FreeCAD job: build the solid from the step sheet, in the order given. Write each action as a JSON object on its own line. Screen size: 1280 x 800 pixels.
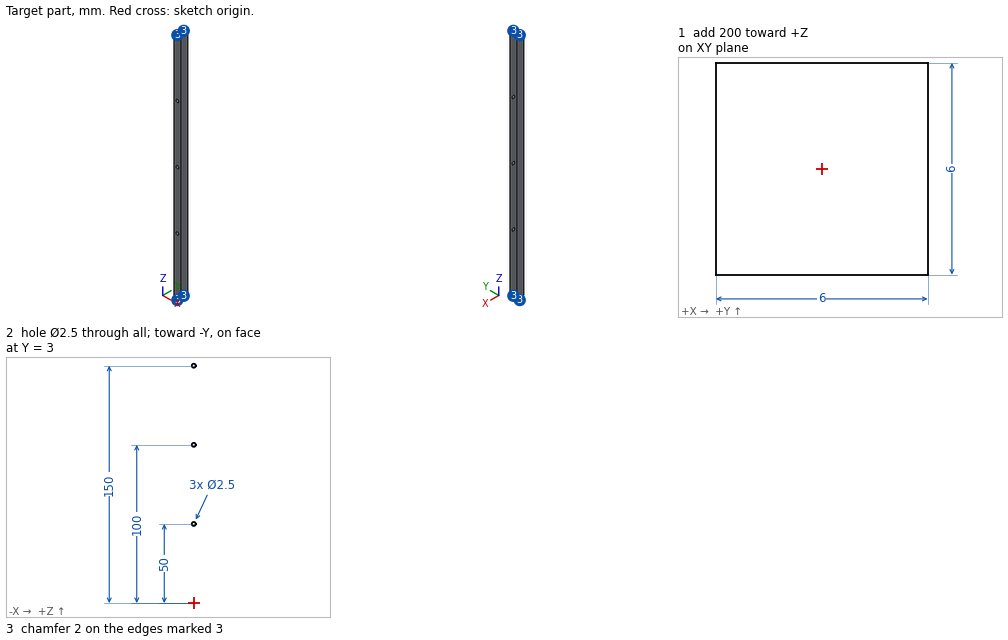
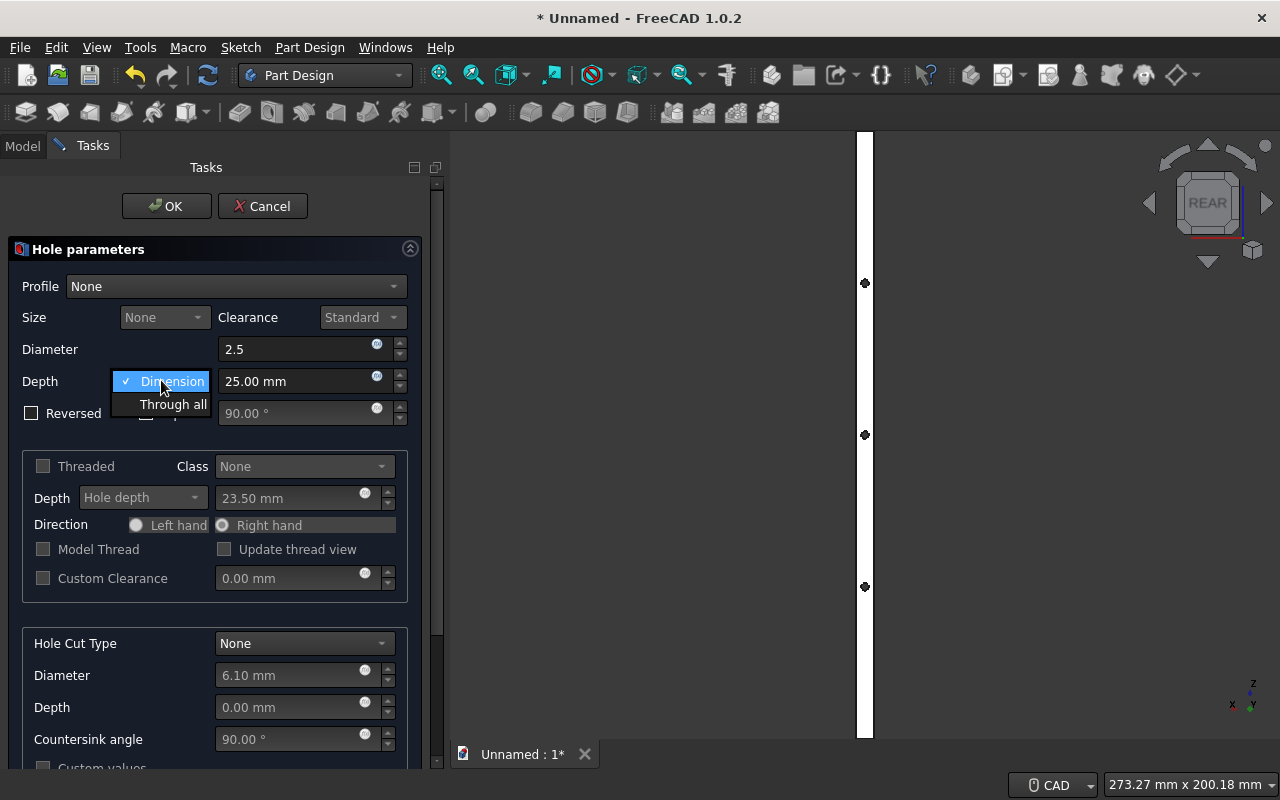
{"action": "left_click", "coordinate": [160, 404]}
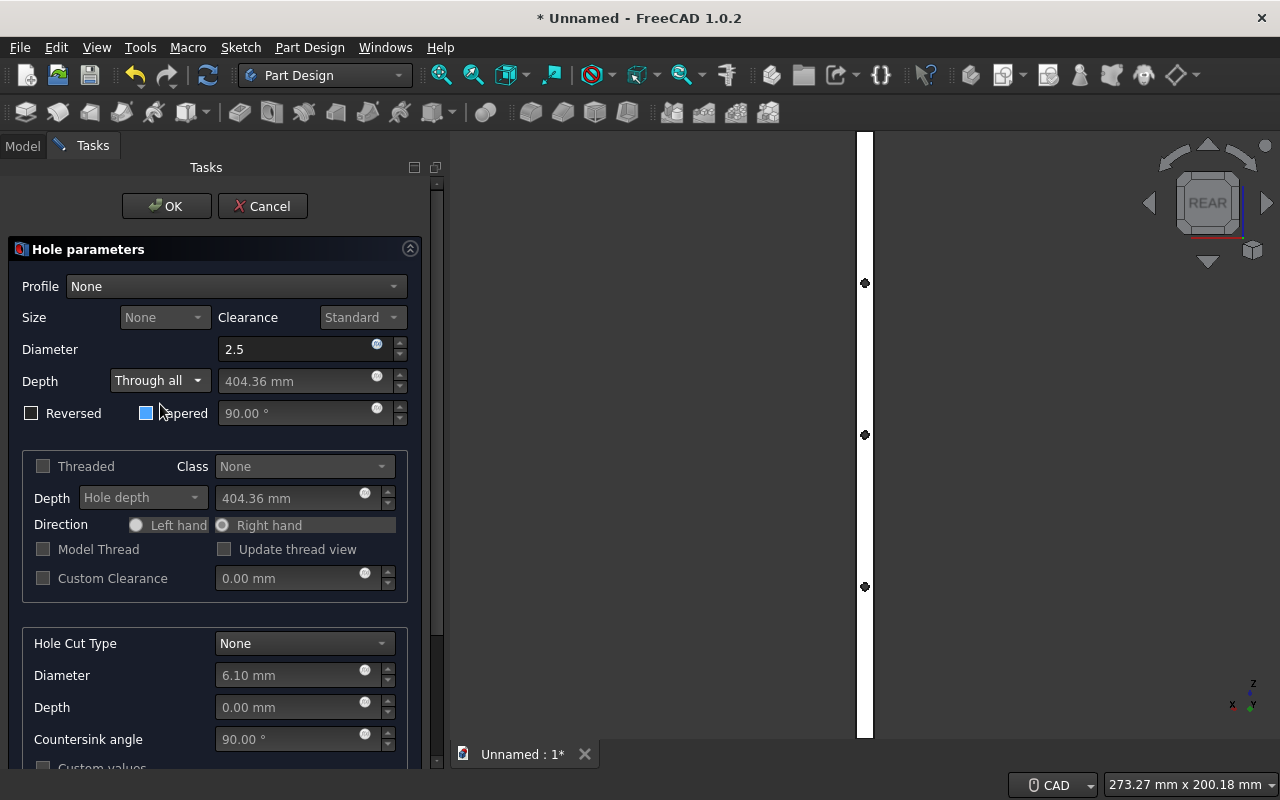
{"action": "left_click", "coordinate": [167, 206]}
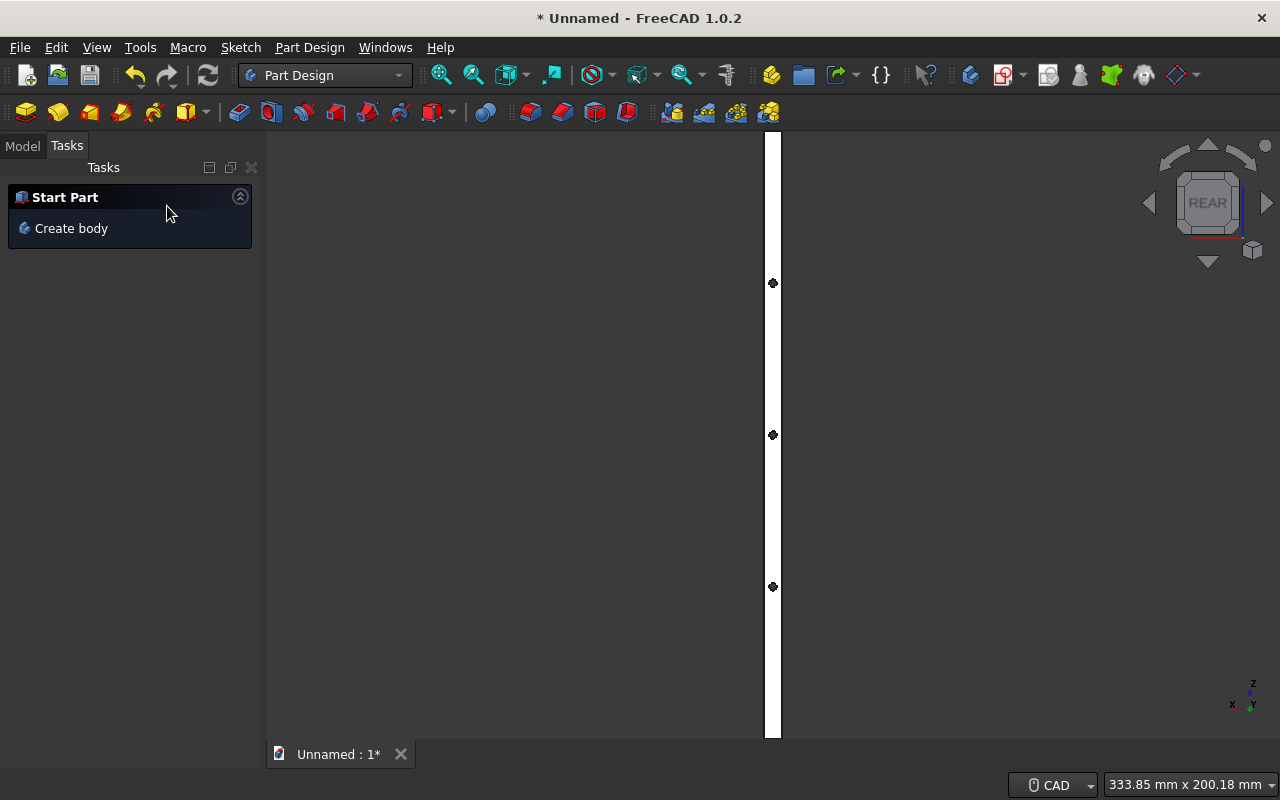
{"action": "left_click", "coordinate": [442, 76]}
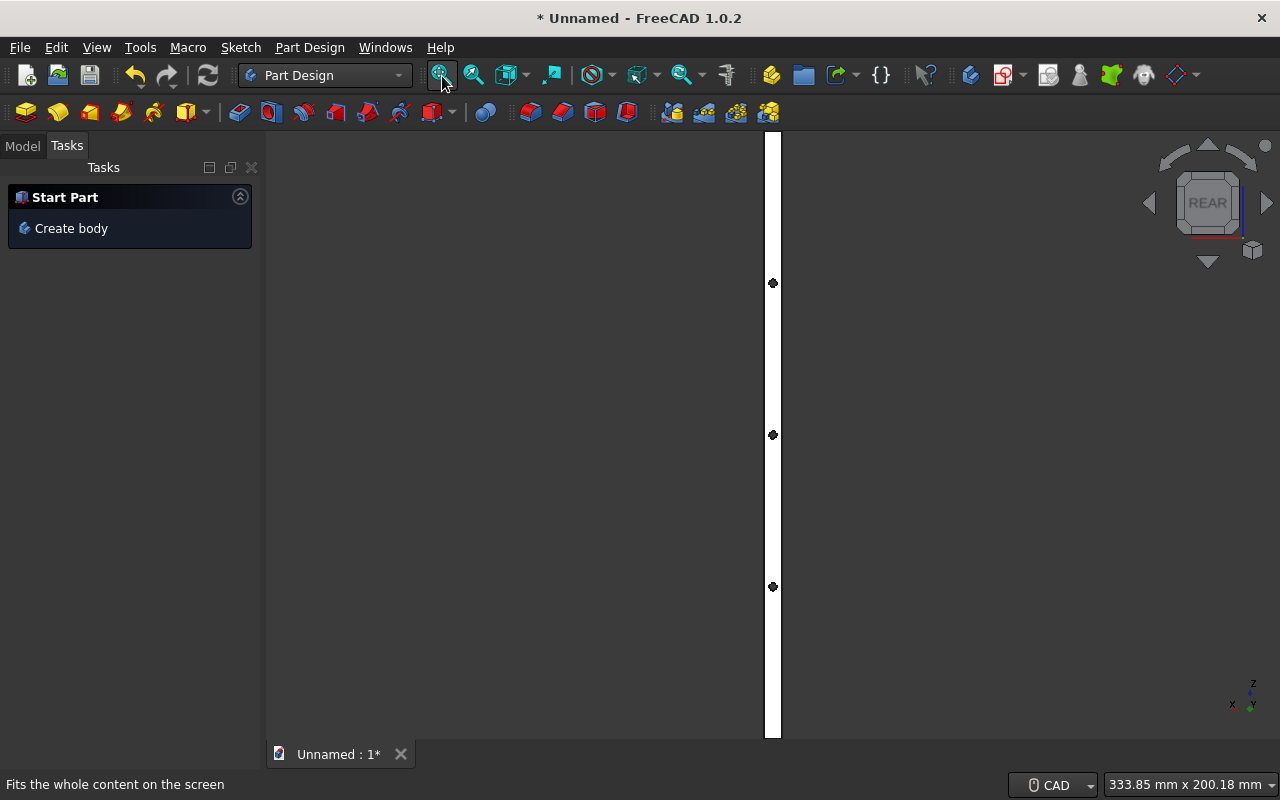
{"action": "key", "text": "0"}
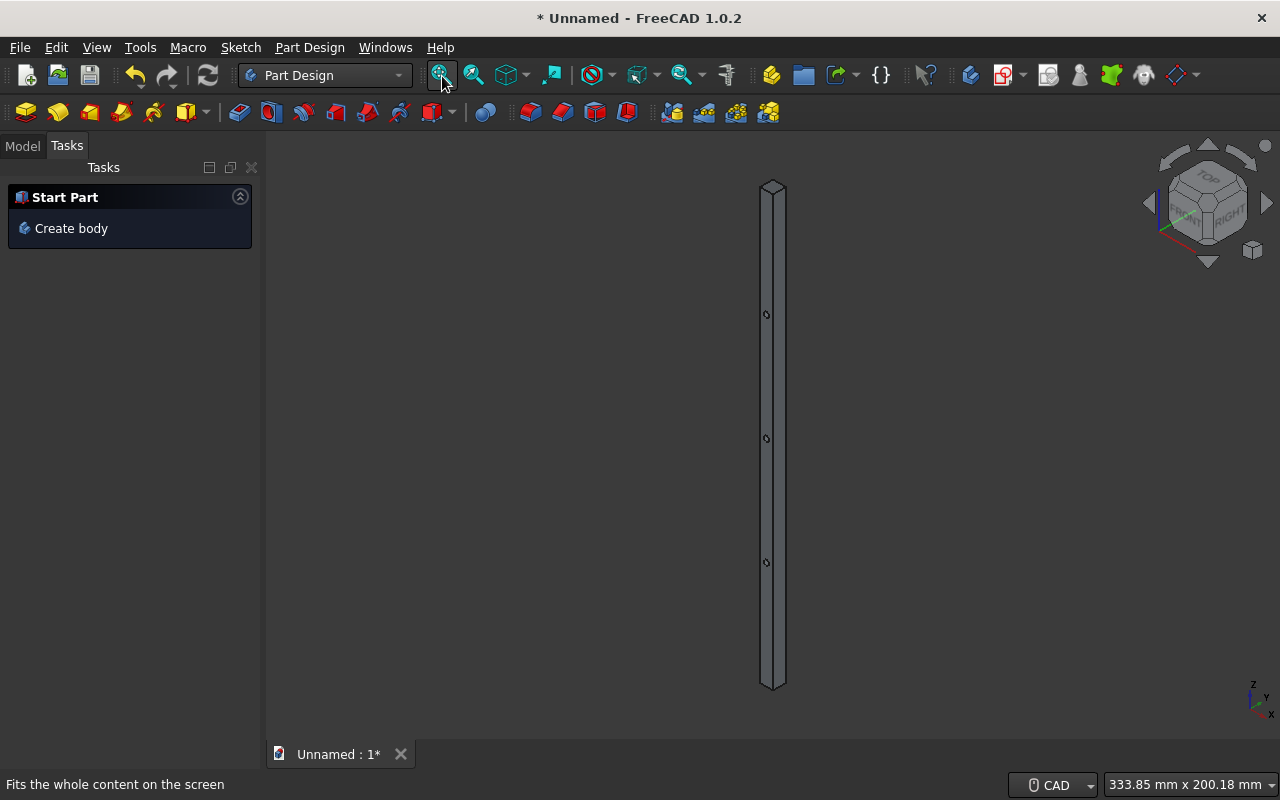
{"action": "left_click", "coordinate": [767, 190]}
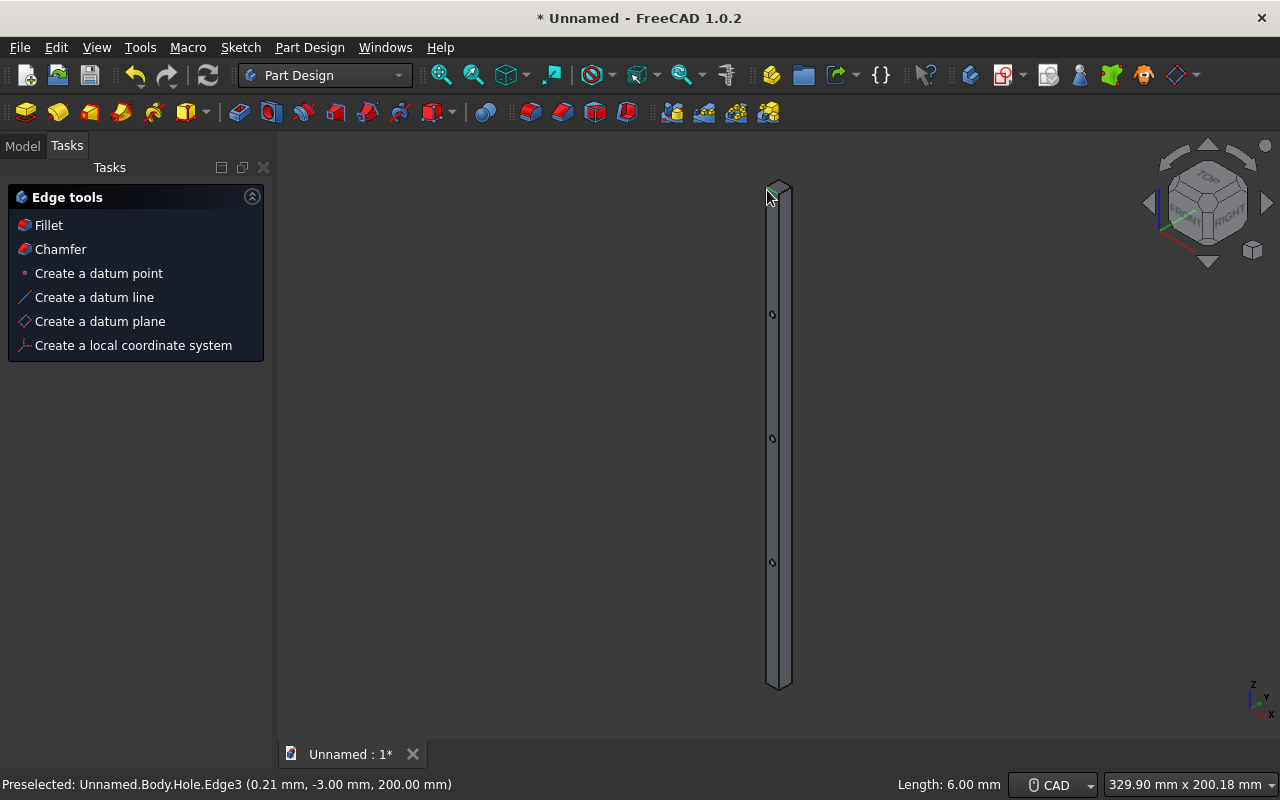
{"action": "scroll", "coordinate": [773, 686], "scroll_direction": "up", "scroll_amount": 4}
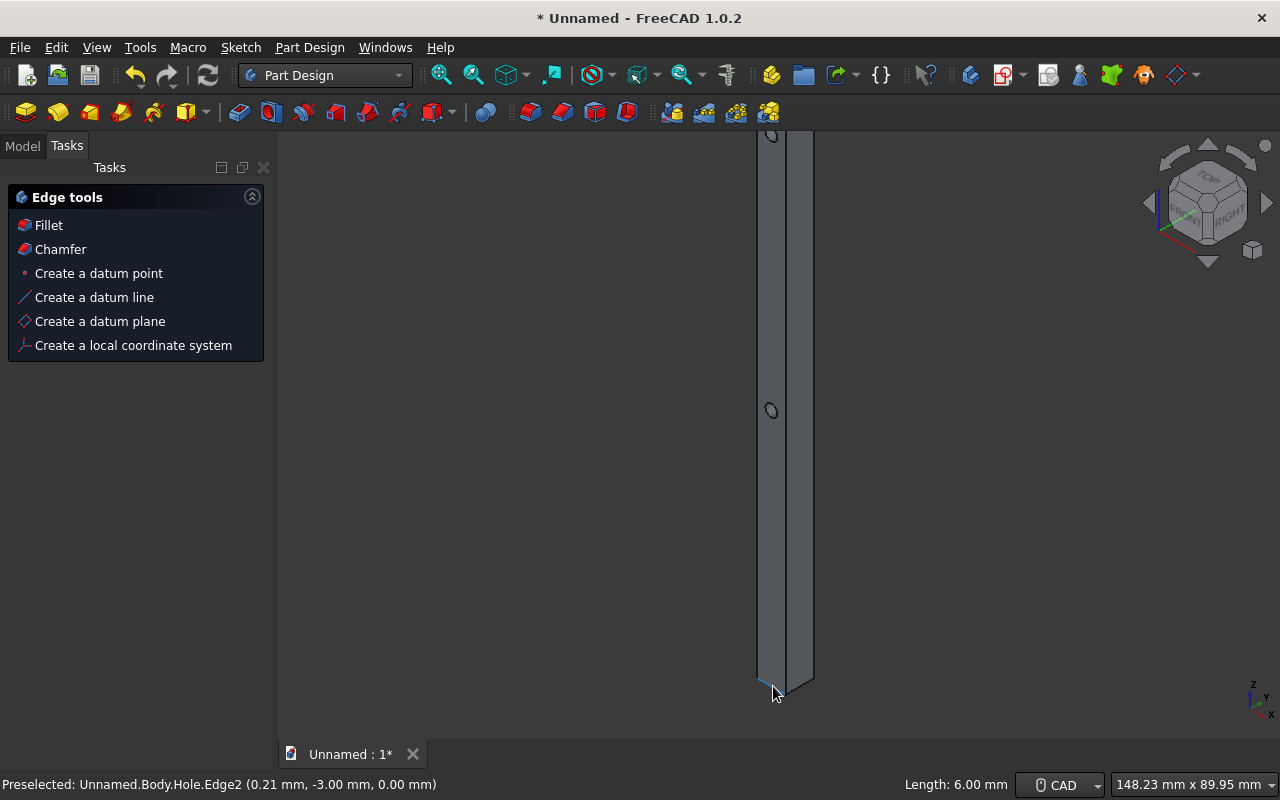
{"action": "left_click", "coordinate": [442, 76]}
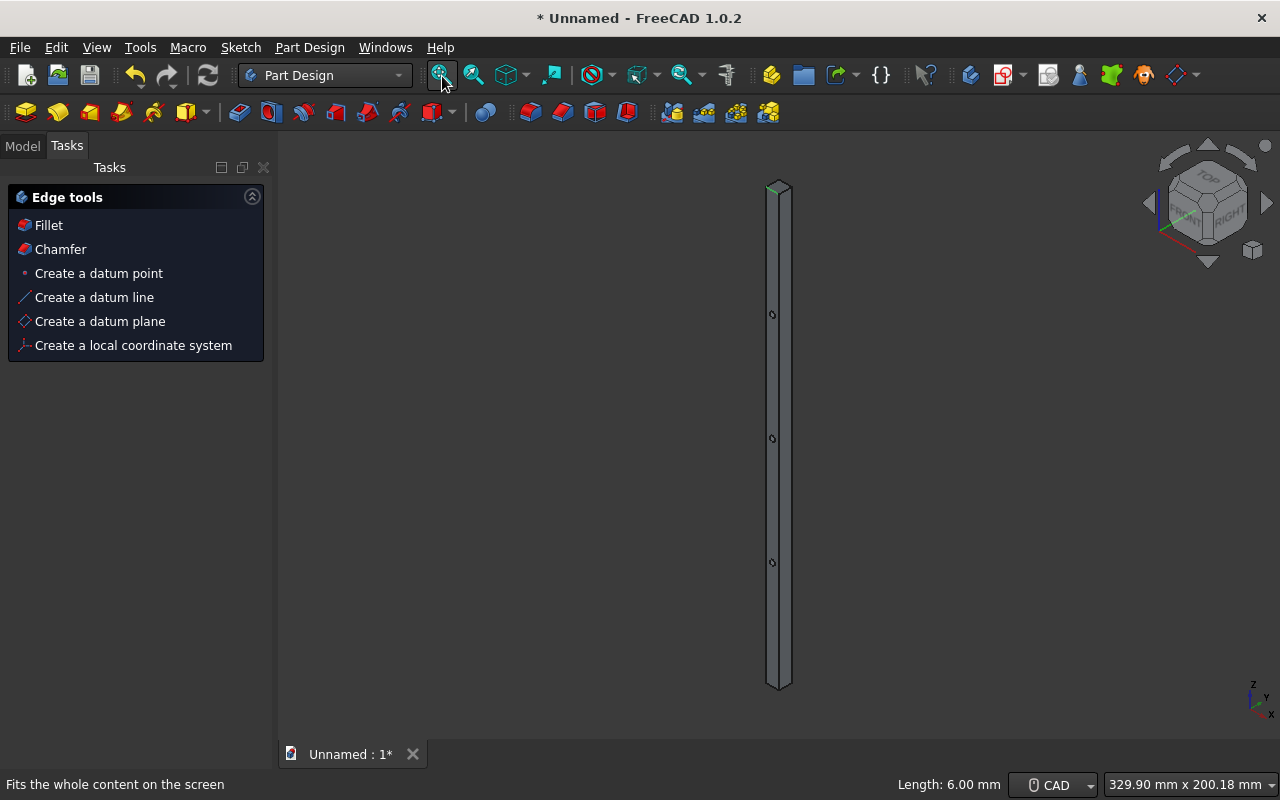
{"action": "key", "text": "2"}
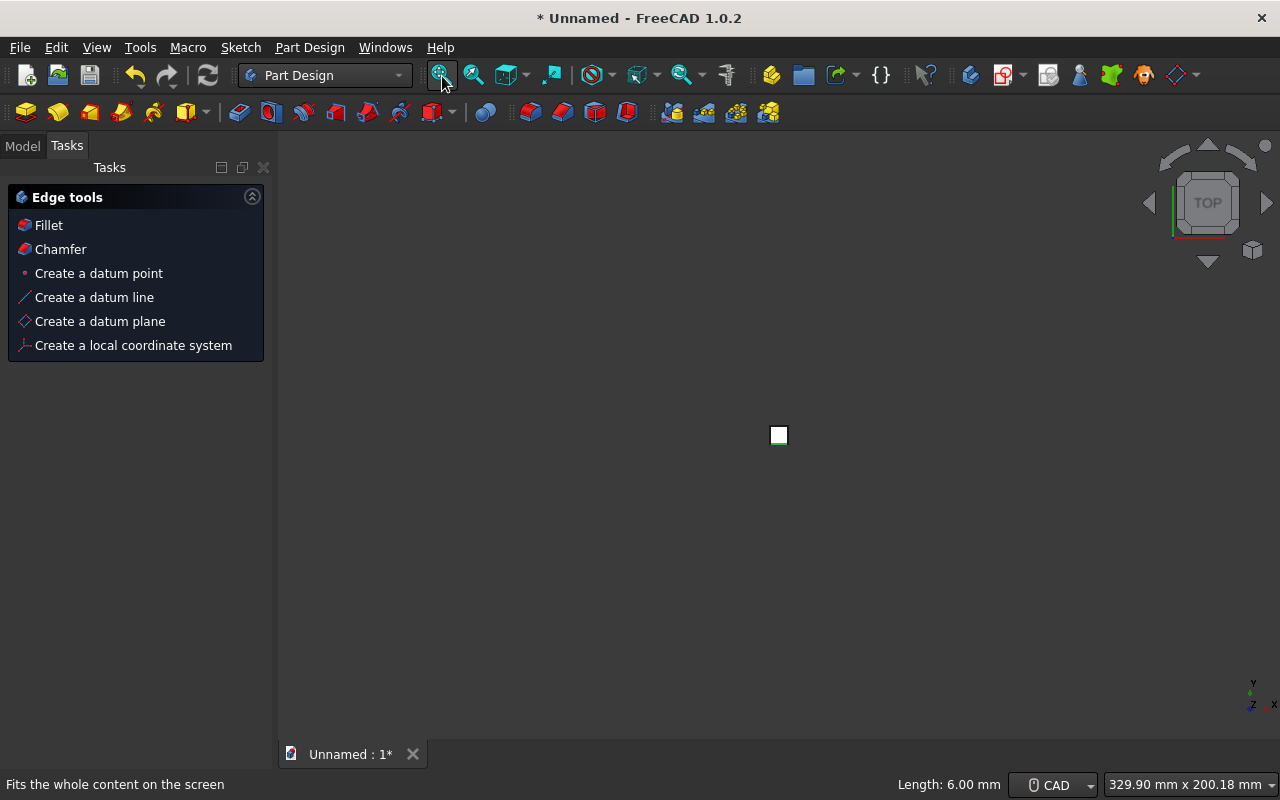
{"action": "left_click", "coordinate": [442, 76]}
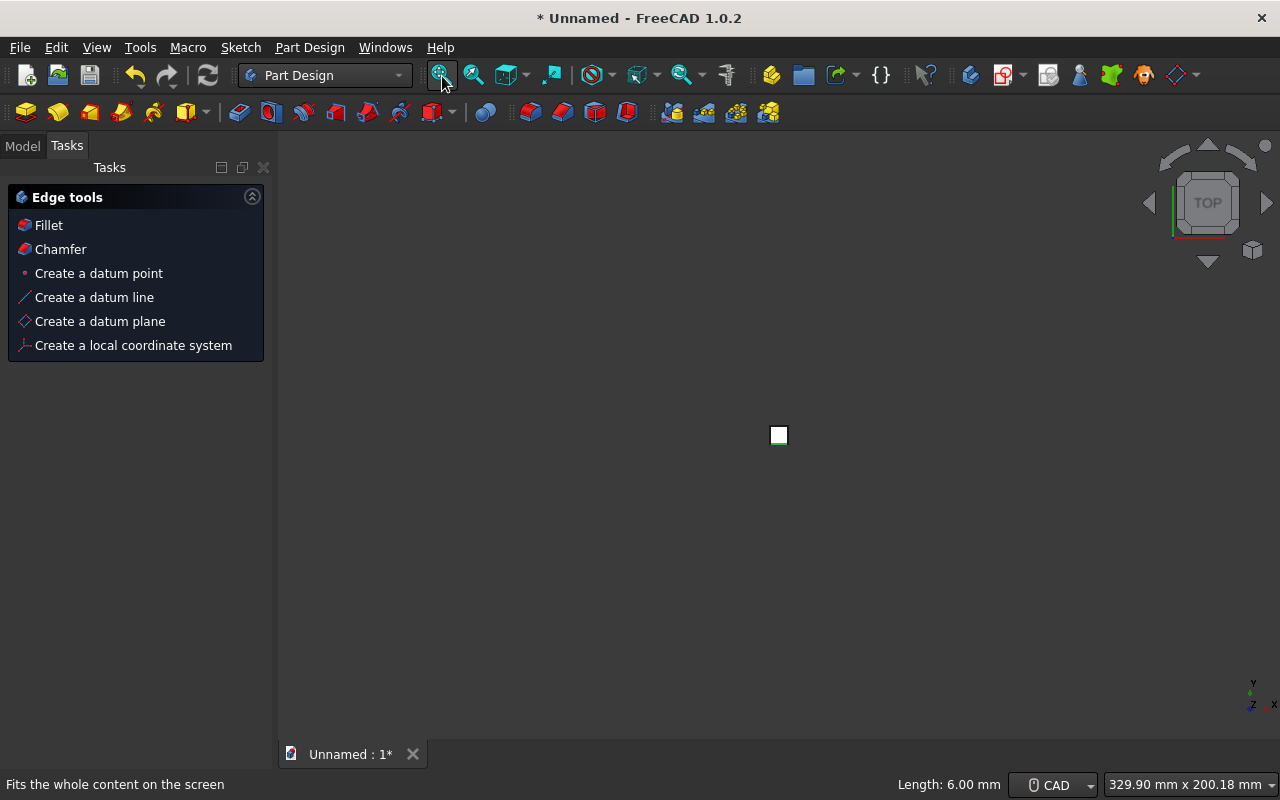
{"action": "left_click", "coordinate": [779, 425], "text": "ctrl"}